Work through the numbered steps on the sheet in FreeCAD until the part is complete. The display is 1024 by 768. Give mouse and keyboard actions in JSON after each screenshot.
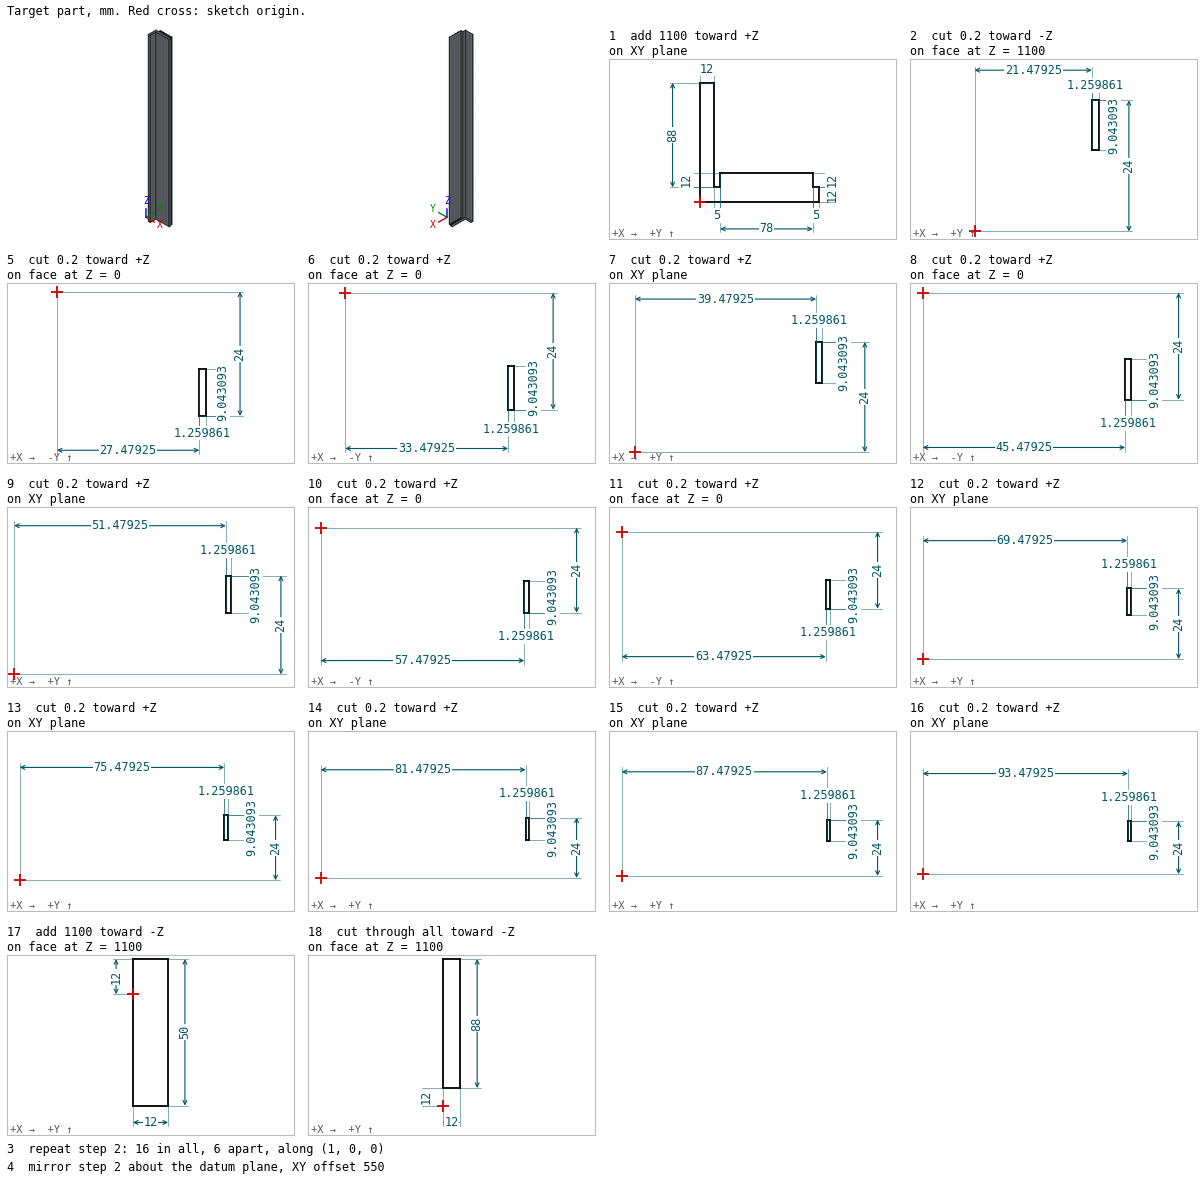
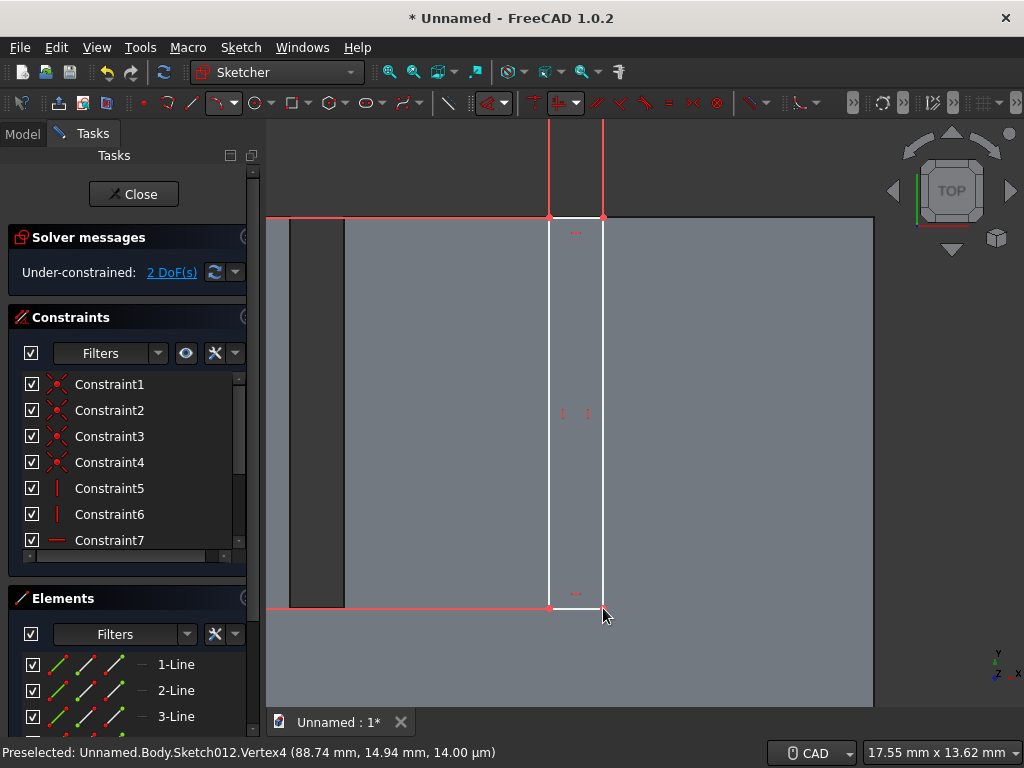
{"action": "left_click", "coordinate": [549, 218]}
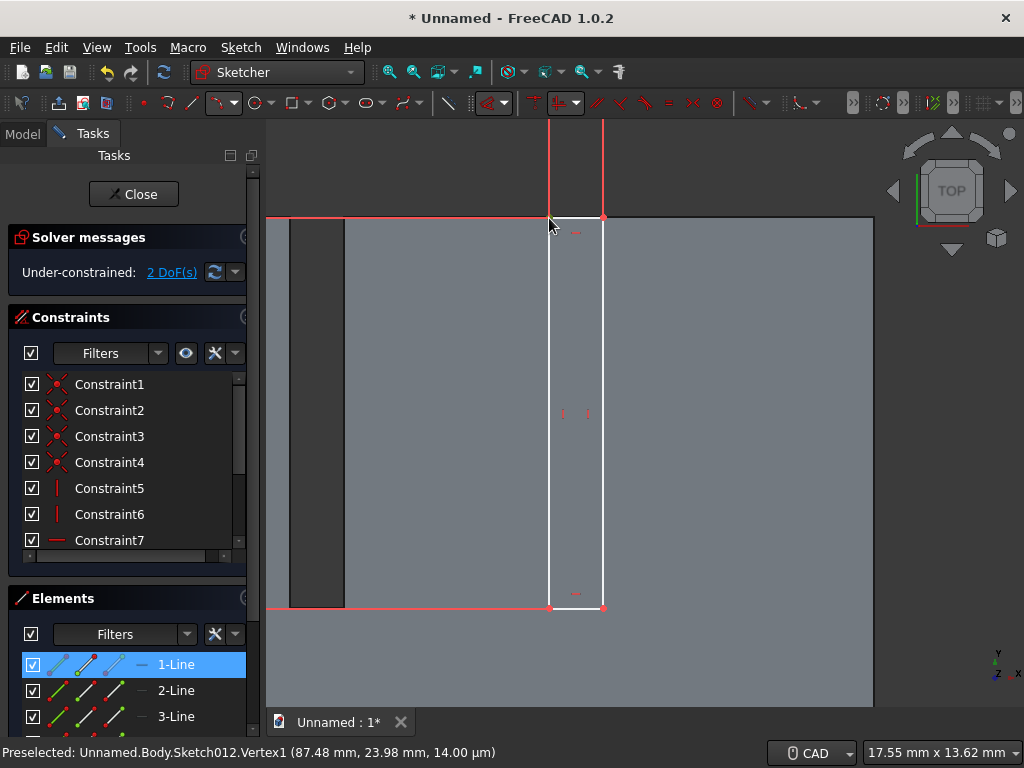
{"action": "left_click", "coordinate": [506, 104]}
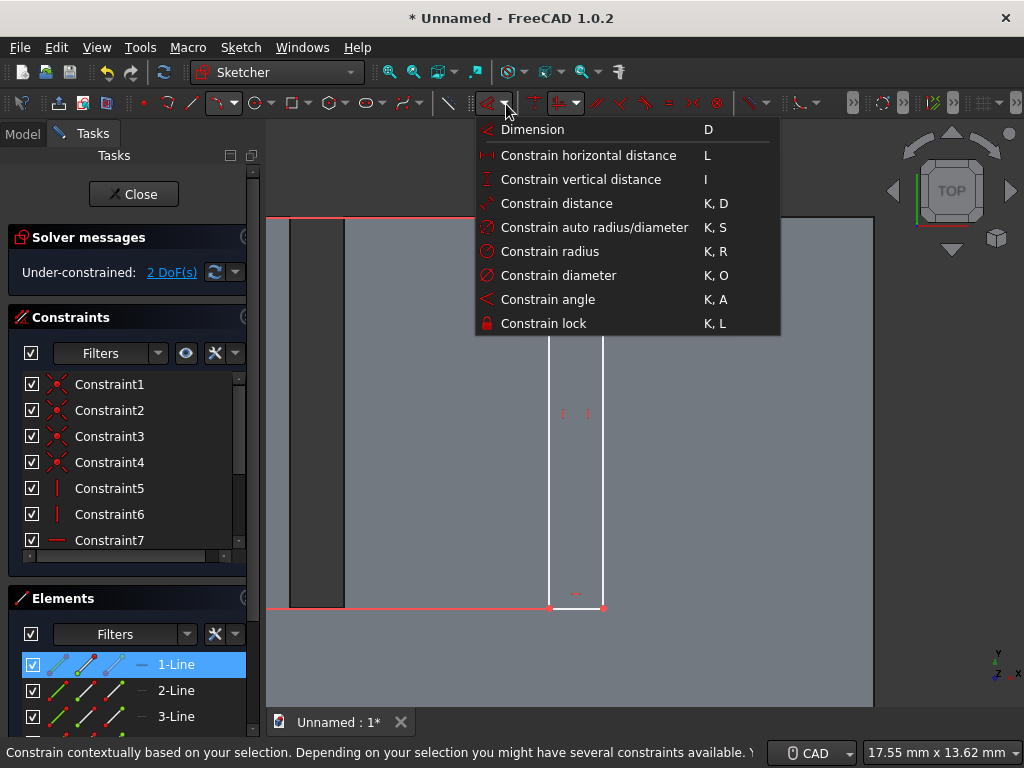
{"action": "left_click", "coordinate": [628, 179]}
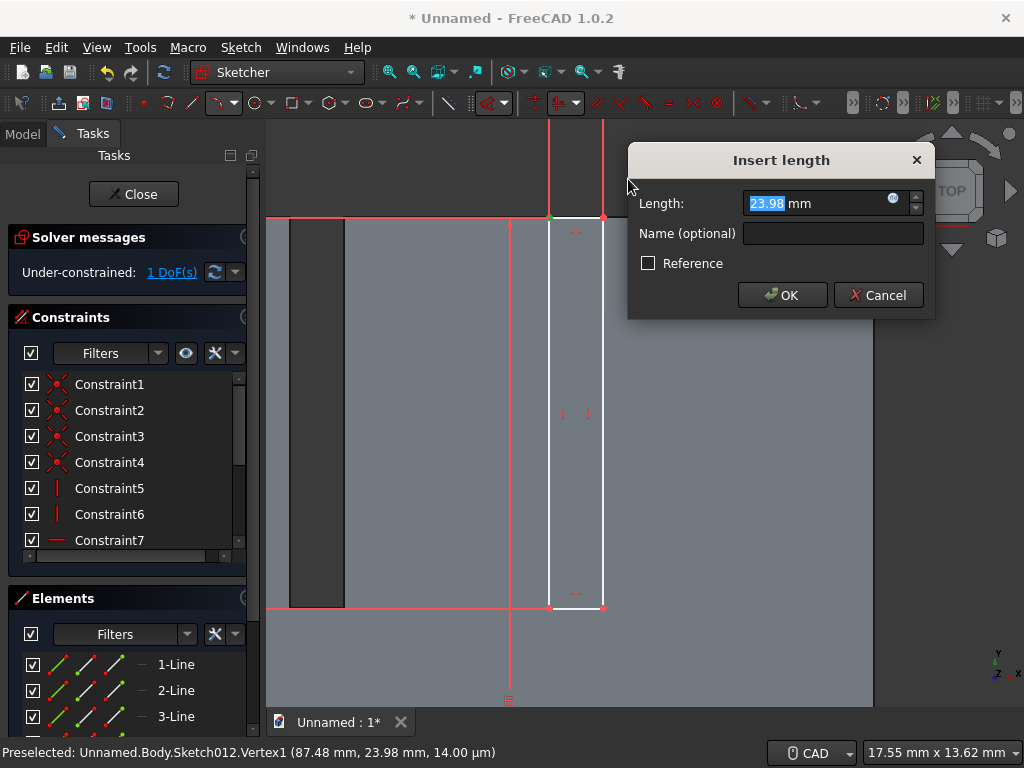
{"action": "type", "text": "24"}
{"action": "key", "text": "Return"}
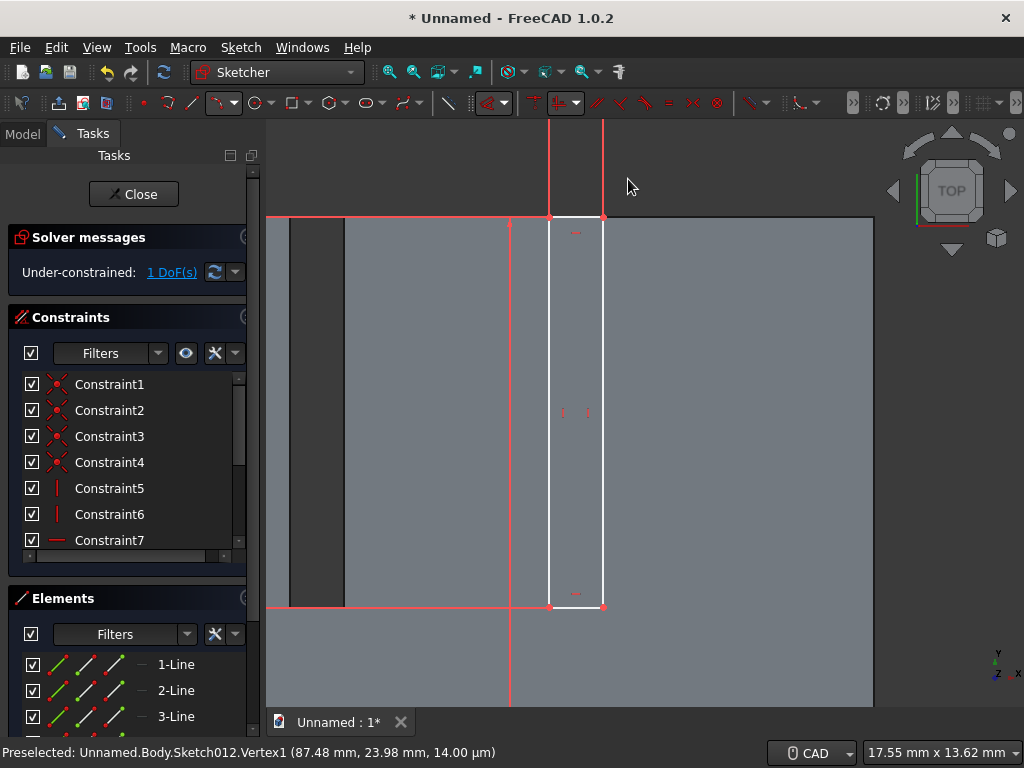
{"action": "left_click", "coordinate": [549, 217]}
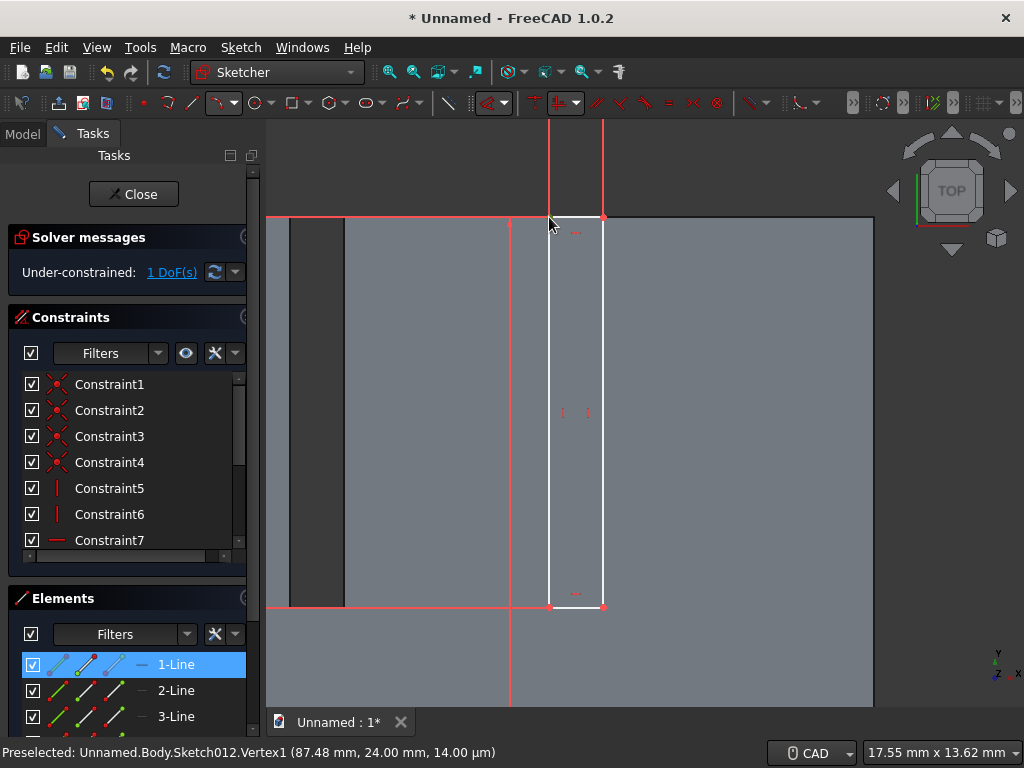
{"action": "key", "text": "l"}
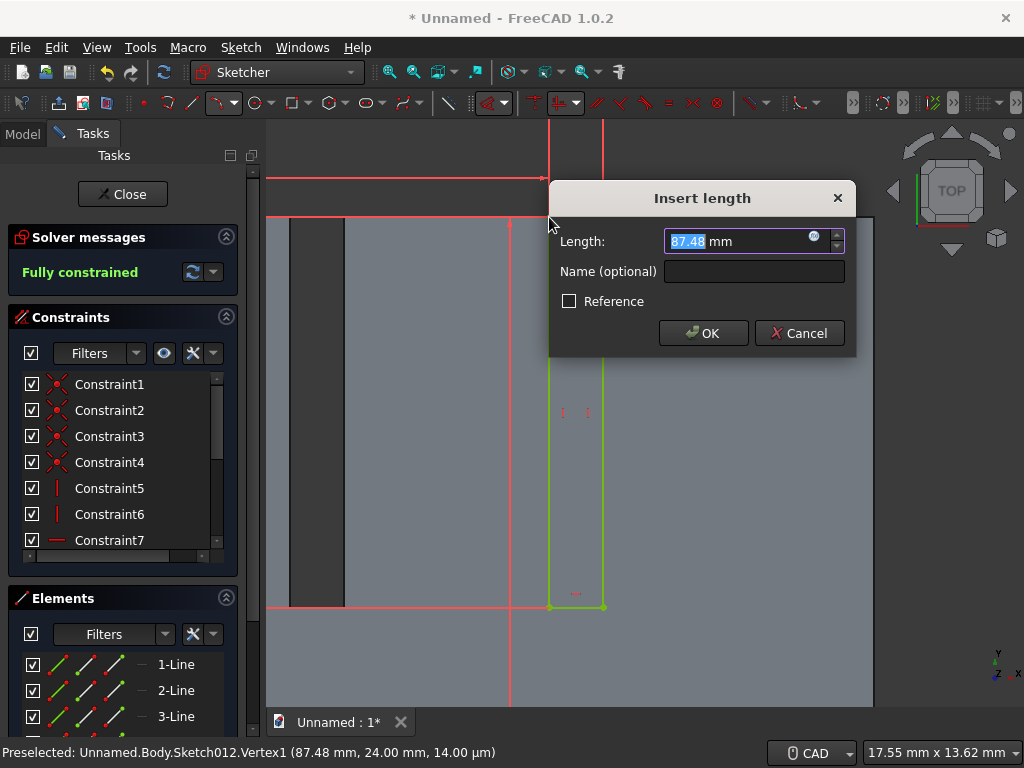
{"action": "type", "text": "87.47925"}
{"action": "key", "text": "Return"}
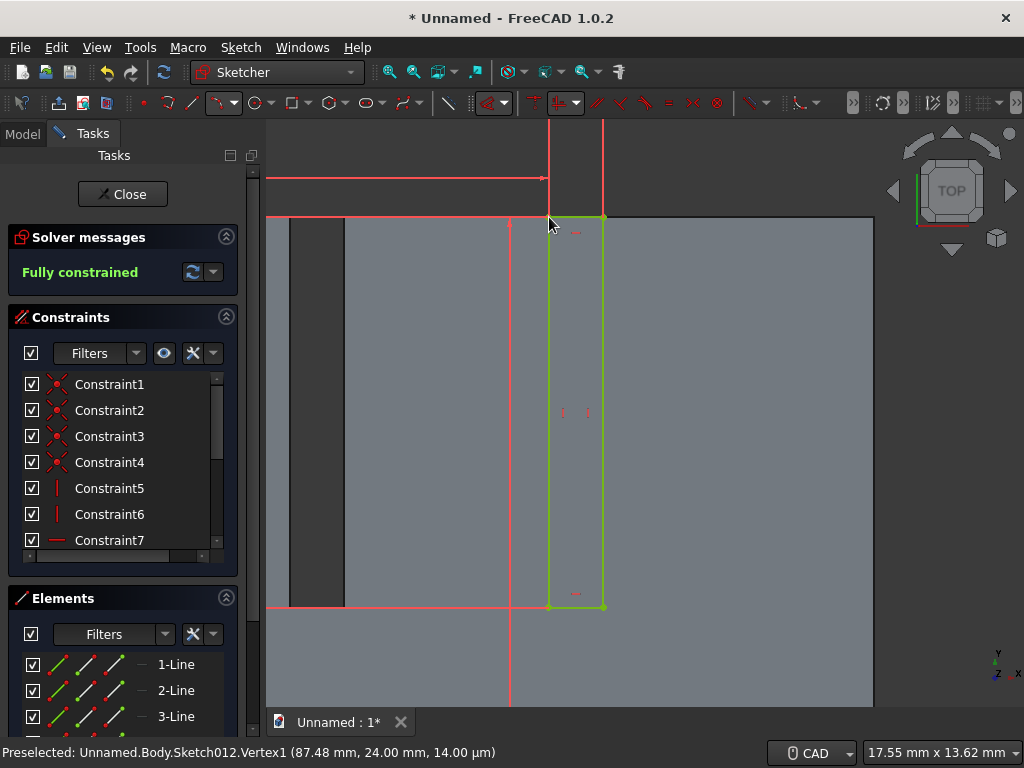
{"action": "left_click", "coordinate": [123, 194]}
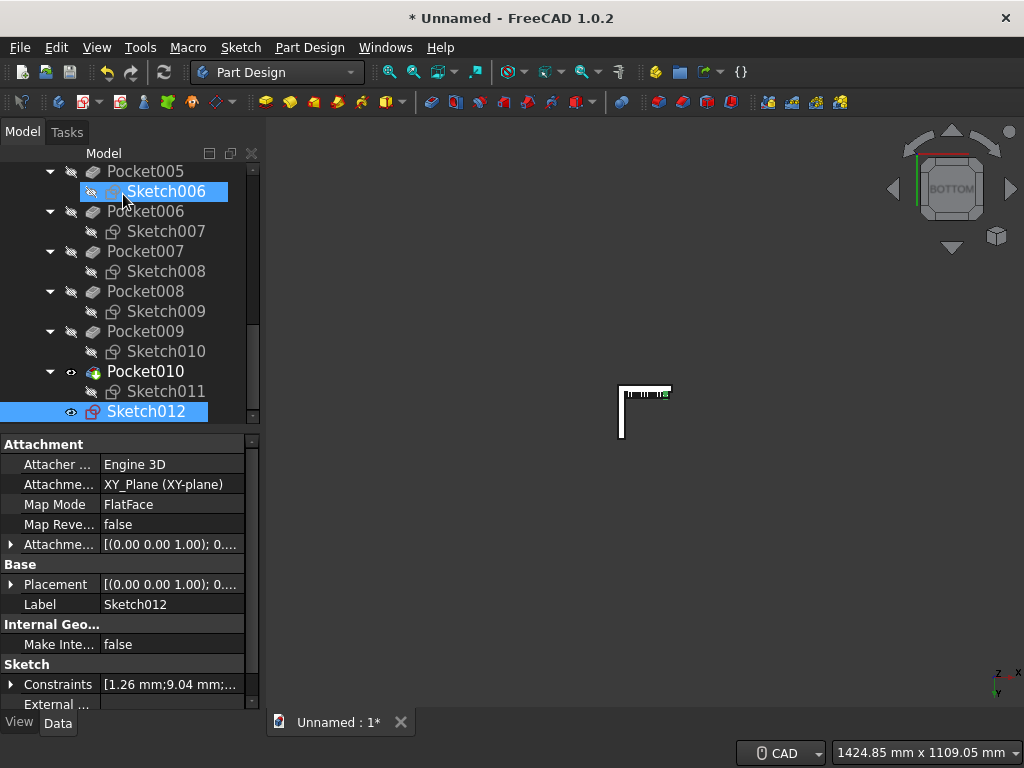
{"action": "left_click", "coordinate": [432, 102]}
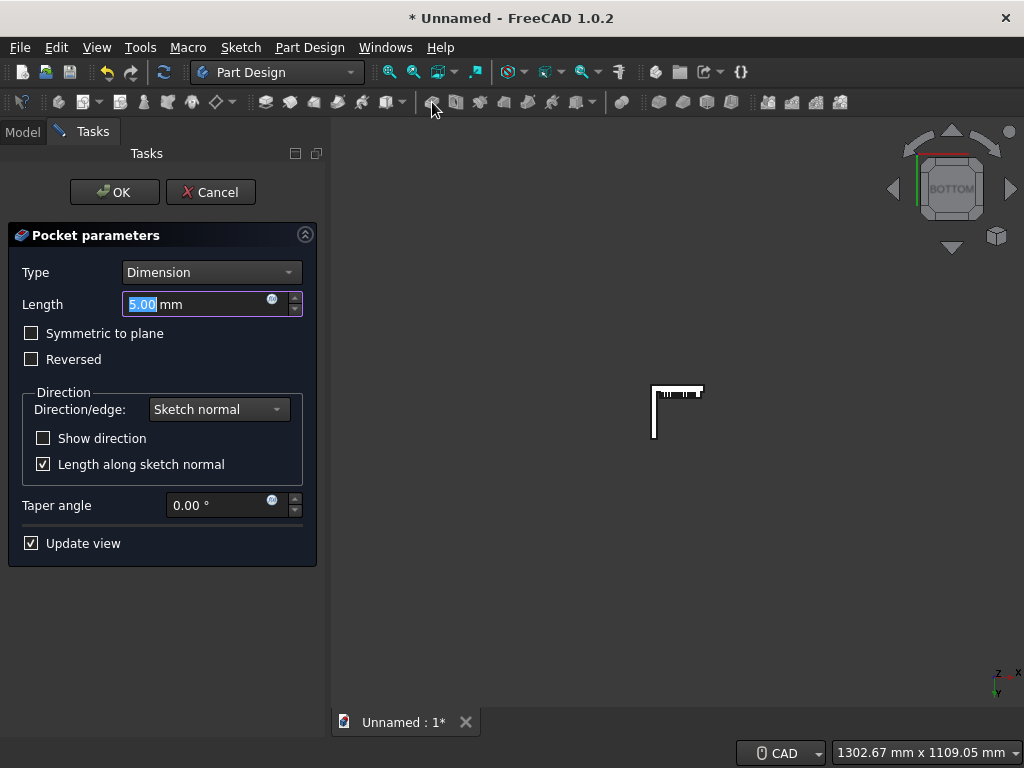
{"action": "type", "text": "0.2"}
{"action": "key", "text": "Tab"}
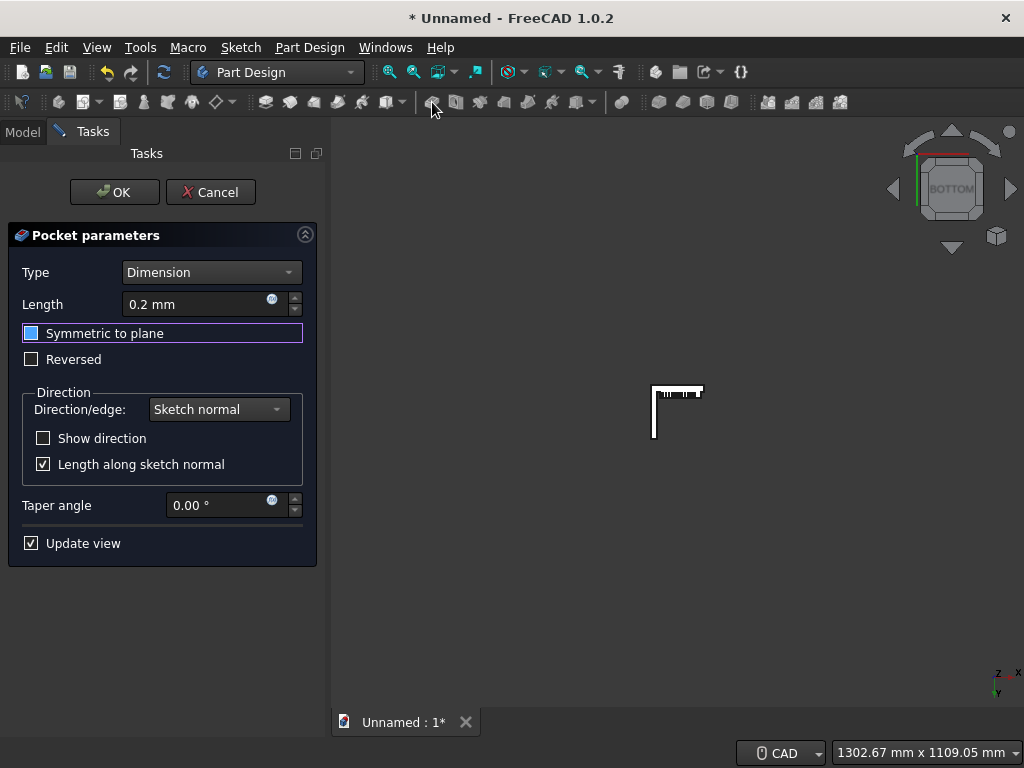
{"action": "left_click", "coordinate": [30, 359]}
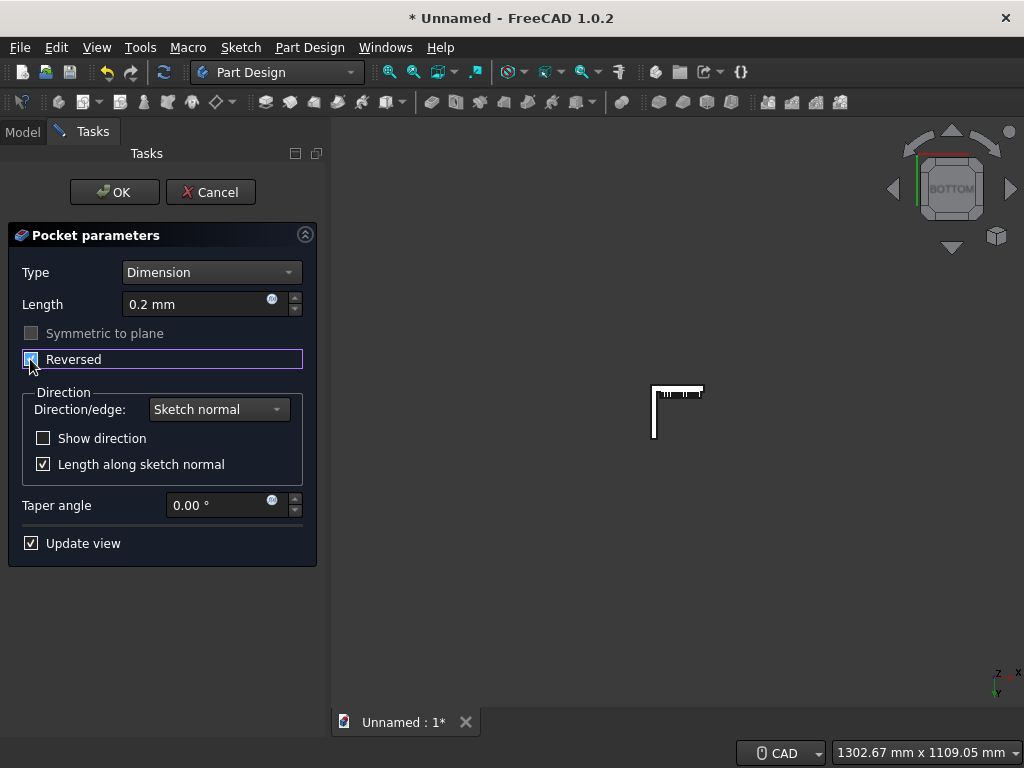
{"action": "left_click", "coordinate": [115, 192]}